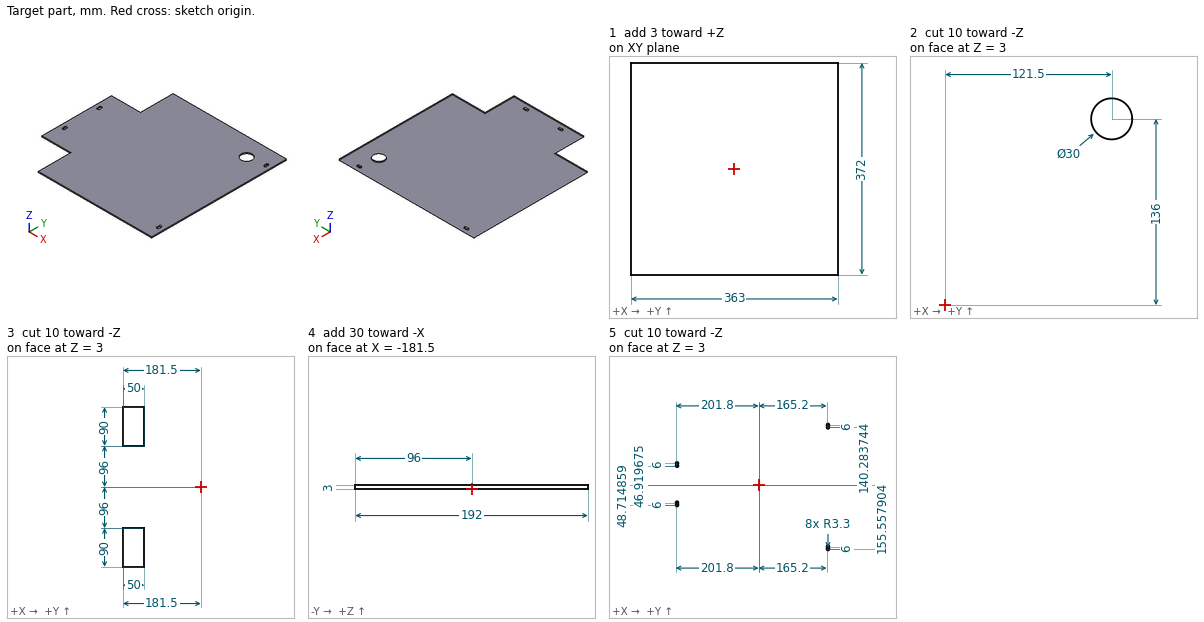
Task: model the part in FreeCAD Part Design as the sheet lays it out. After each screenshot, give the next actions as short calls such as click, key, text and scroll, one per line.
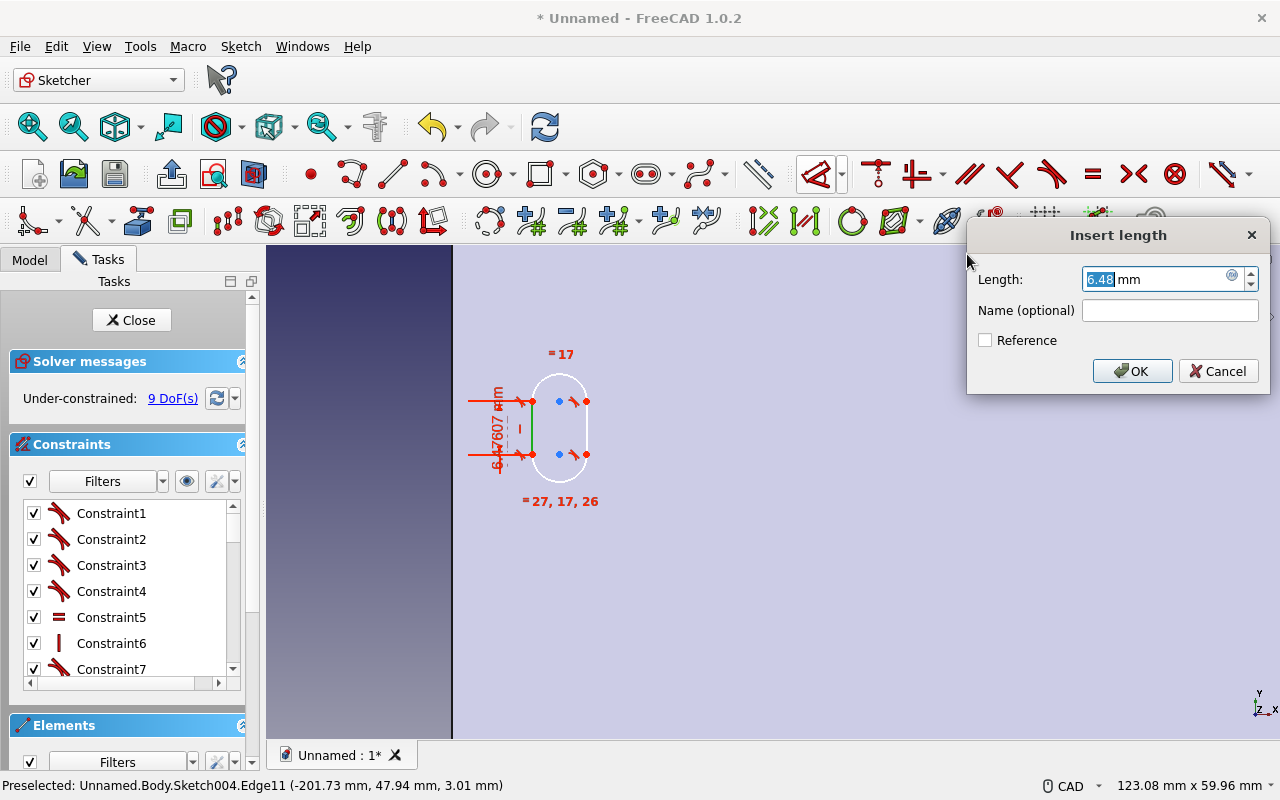
text(6)
key(Return)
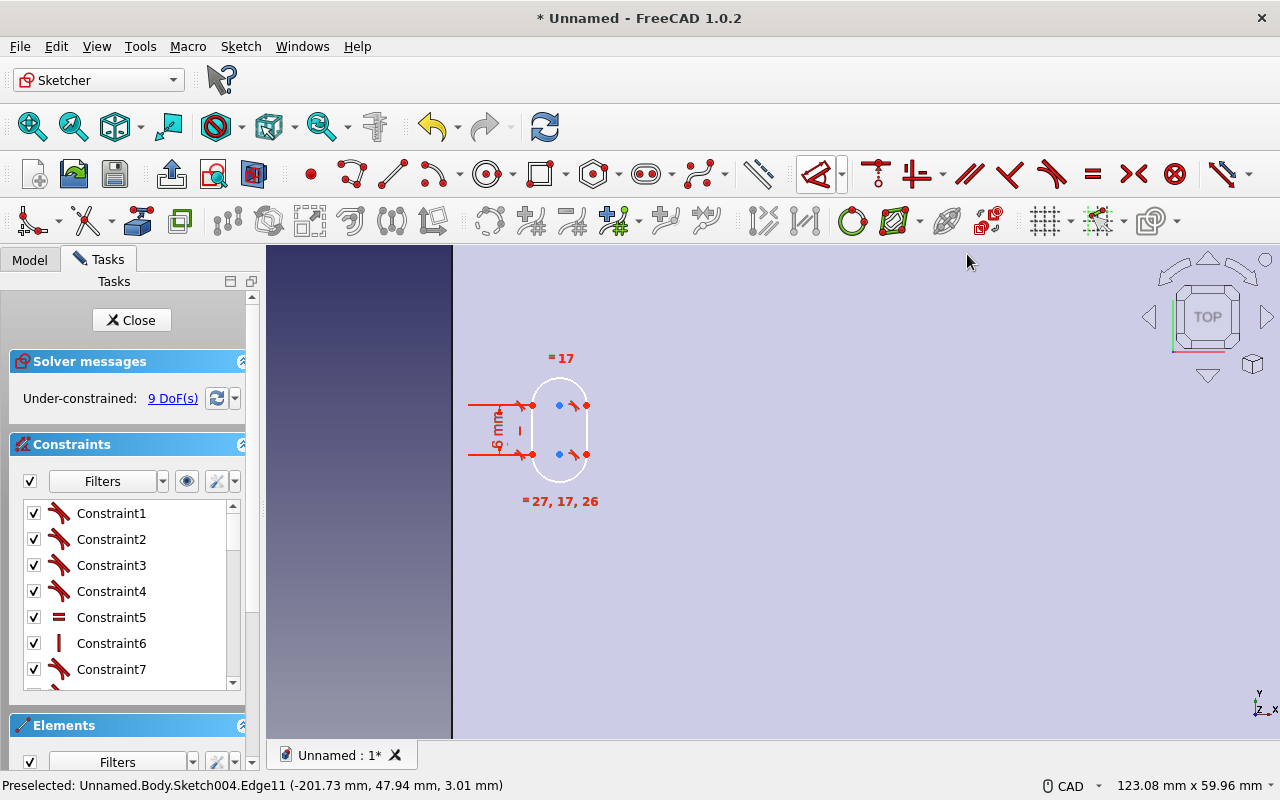
scroll(534, 445, down, 11)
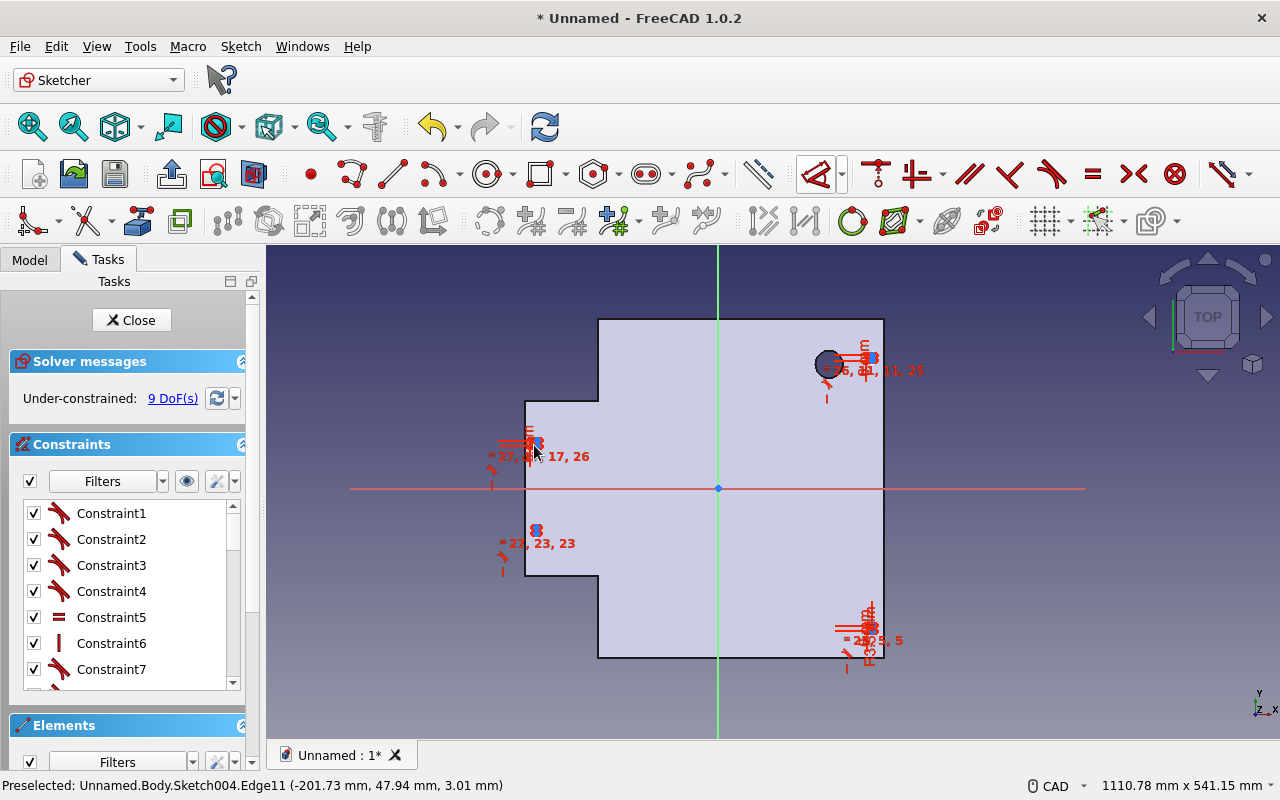
scroll(533, 532, up, 11)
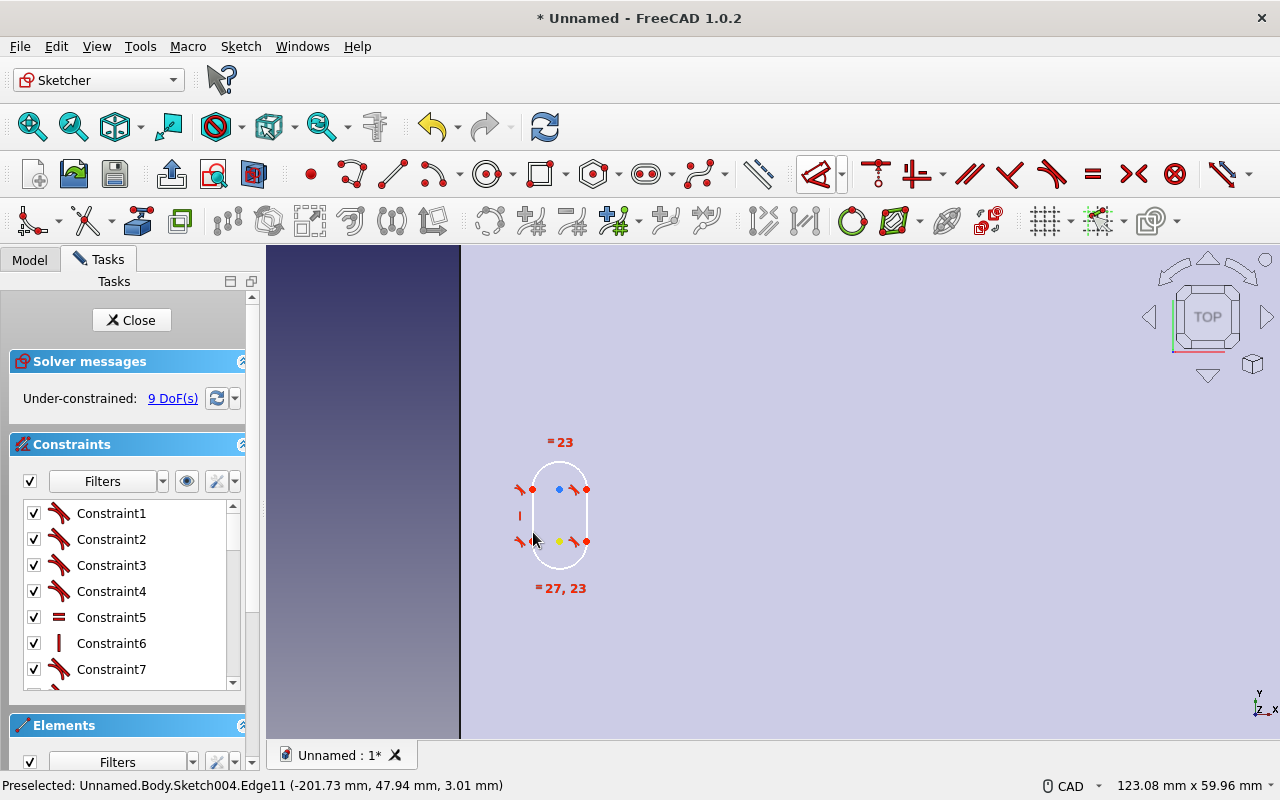
click(533, 526)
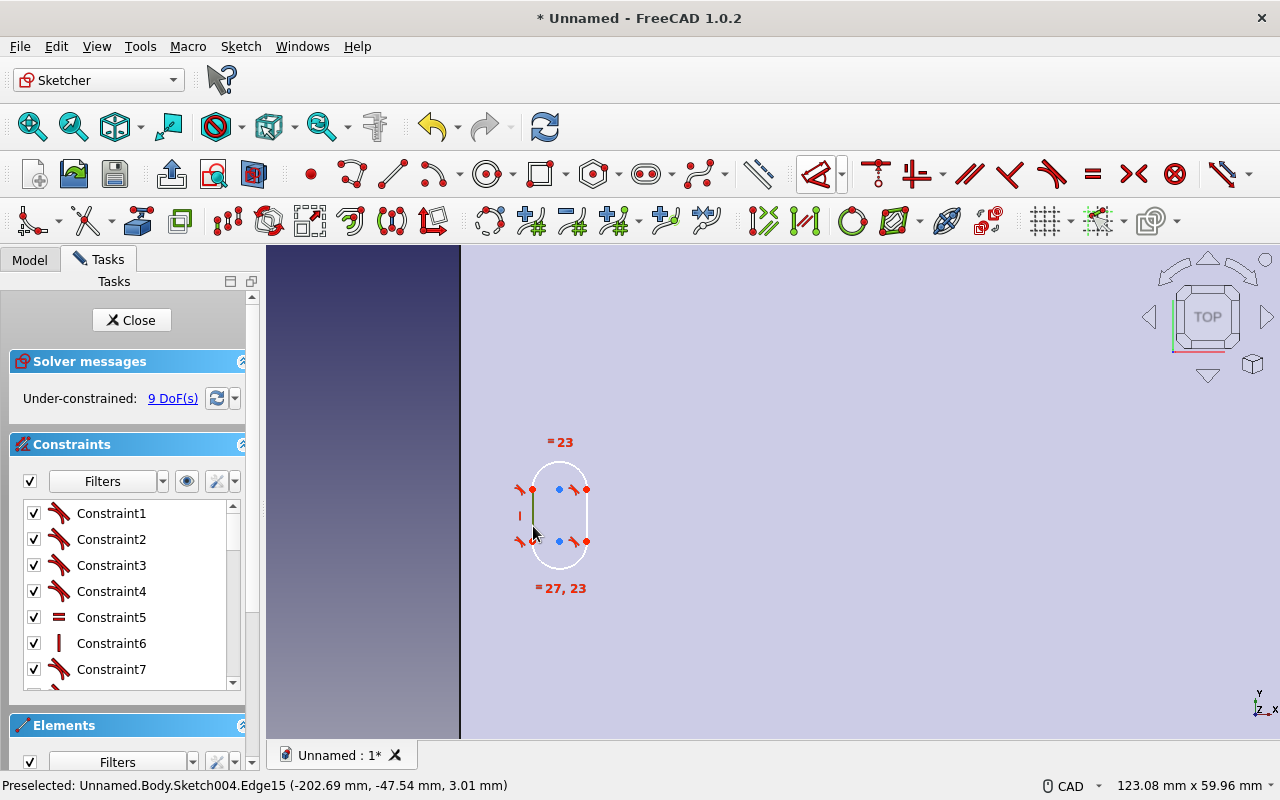
key(i)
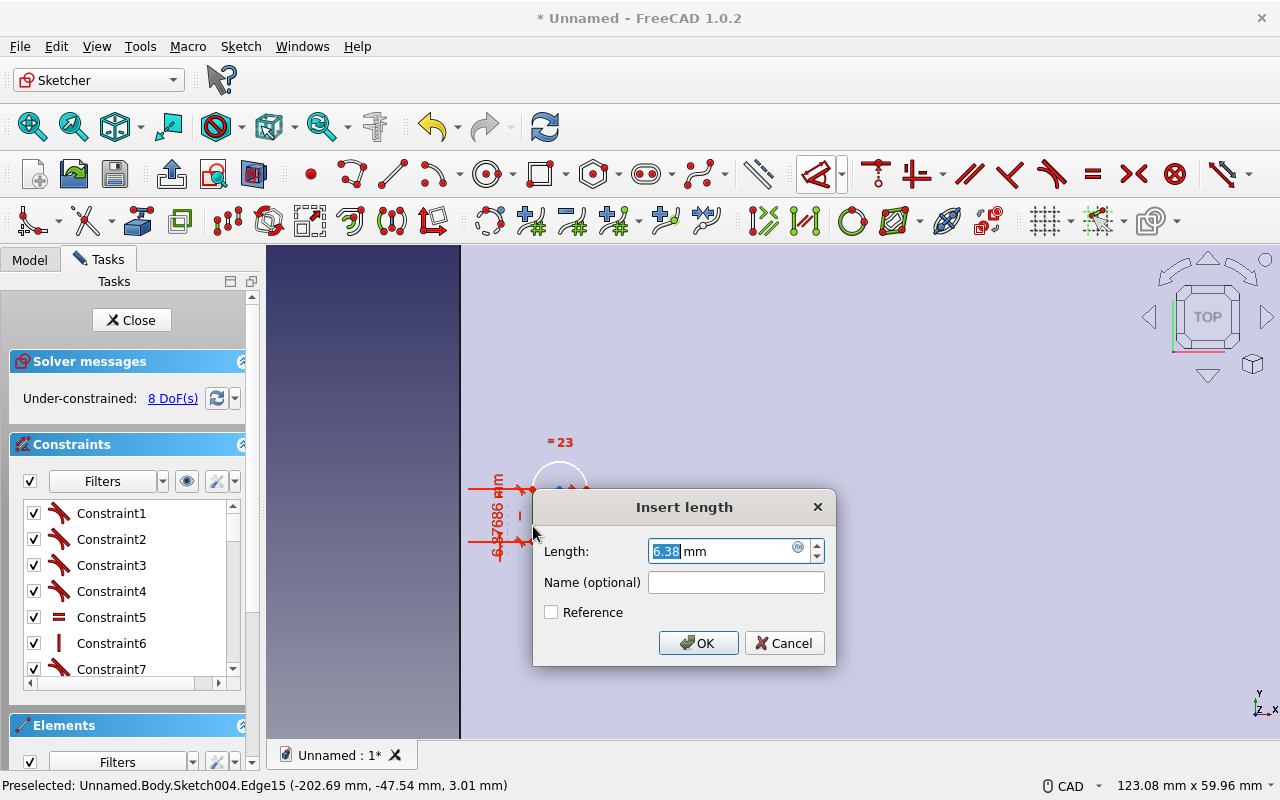
text(6)
key(Return)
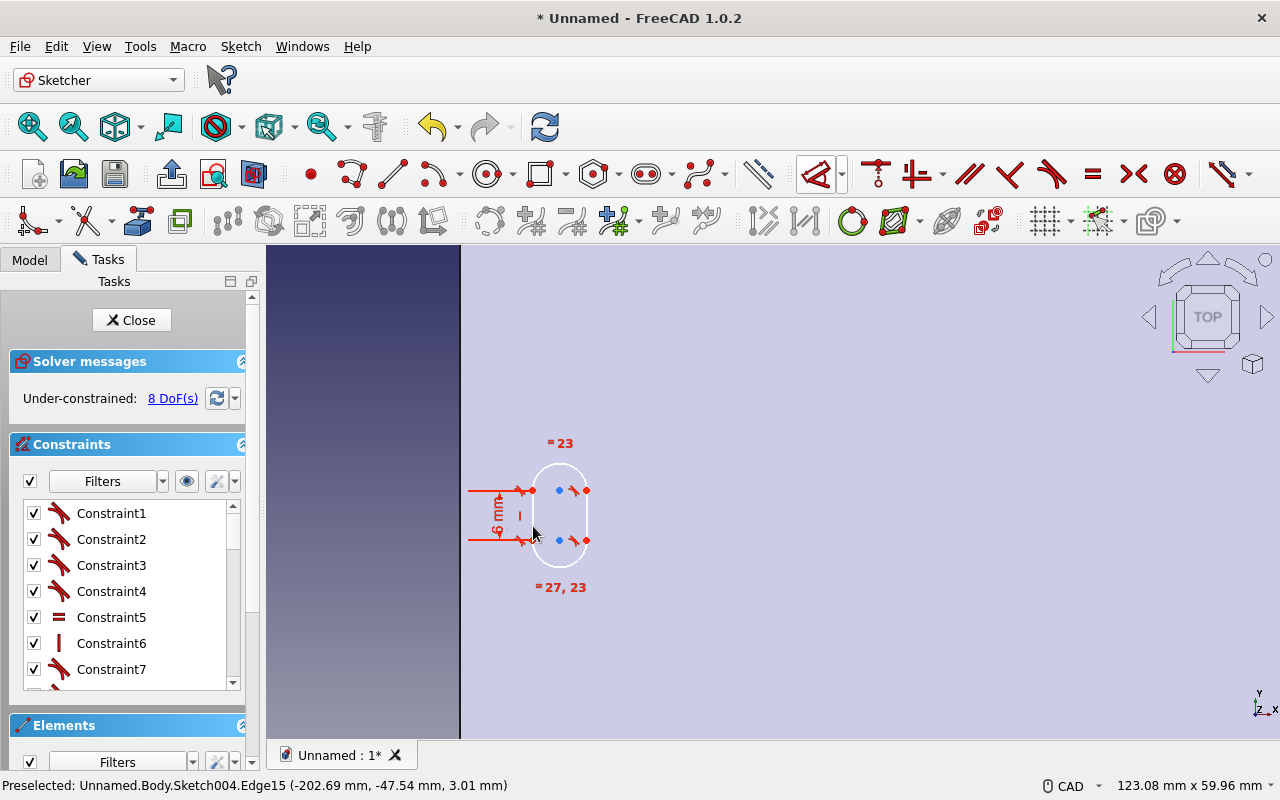
scroll(533, 532, down, 11)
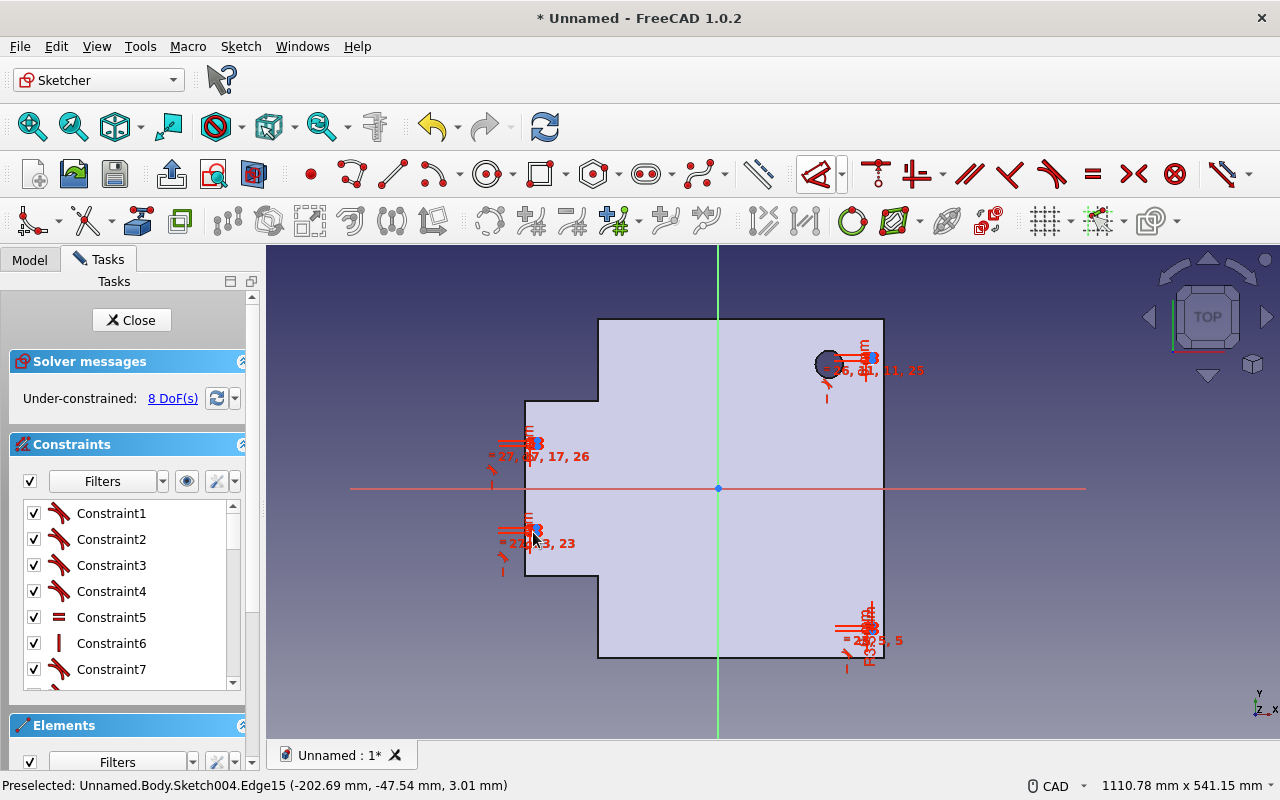
scroll(869, 631, up, 7)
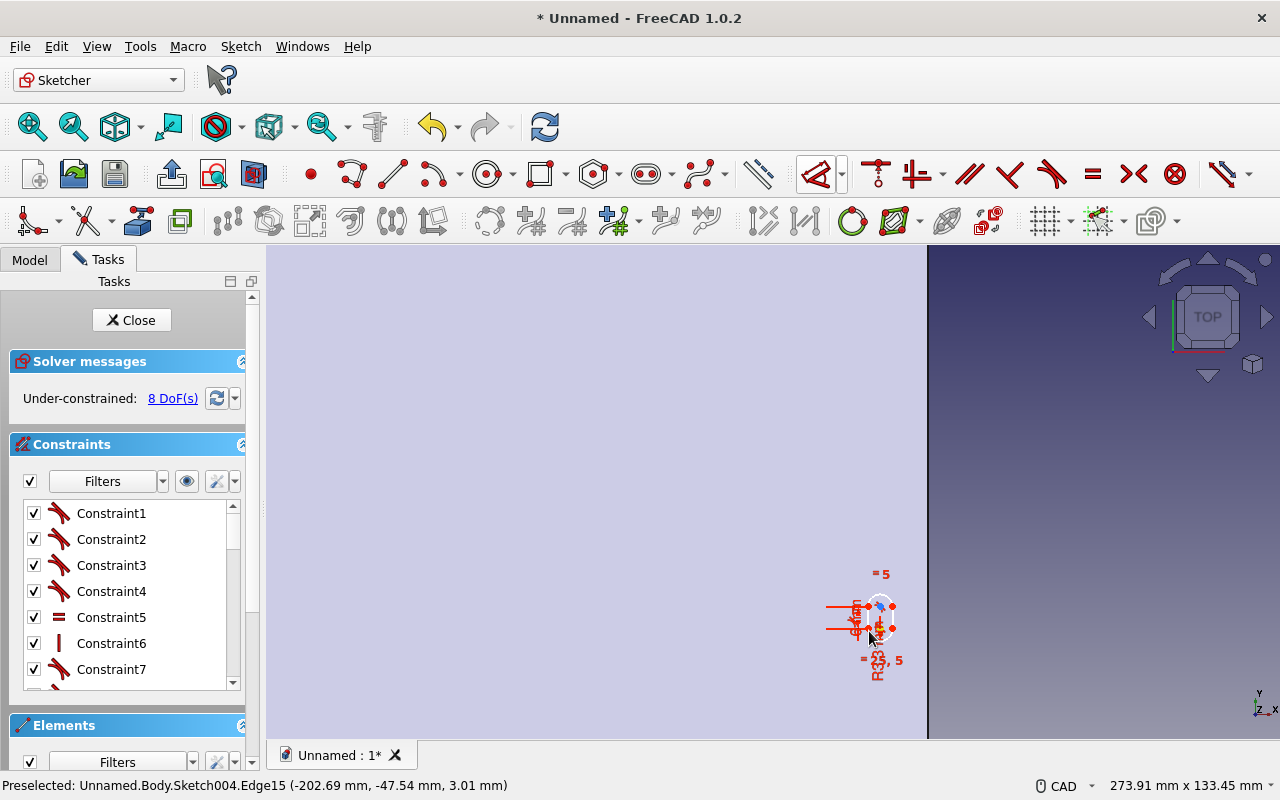
click(868, 629)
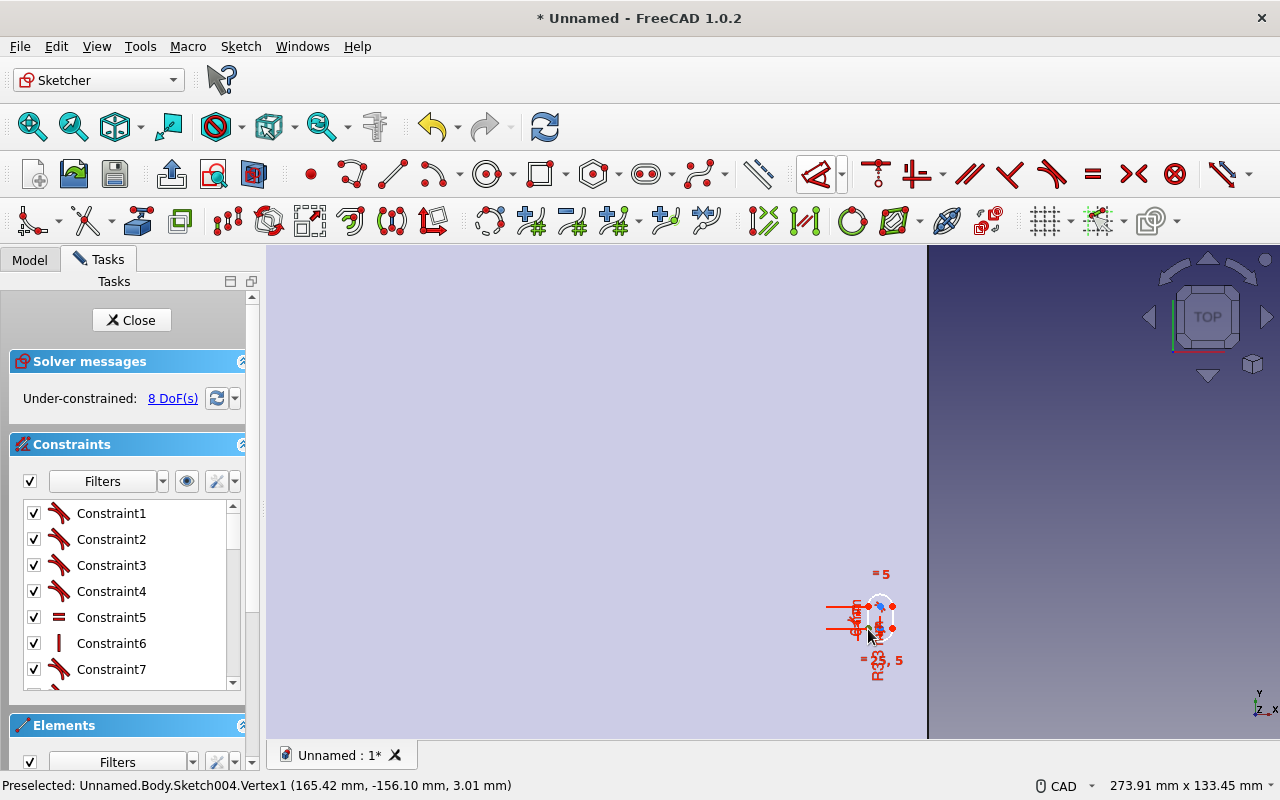
click(842, 174)